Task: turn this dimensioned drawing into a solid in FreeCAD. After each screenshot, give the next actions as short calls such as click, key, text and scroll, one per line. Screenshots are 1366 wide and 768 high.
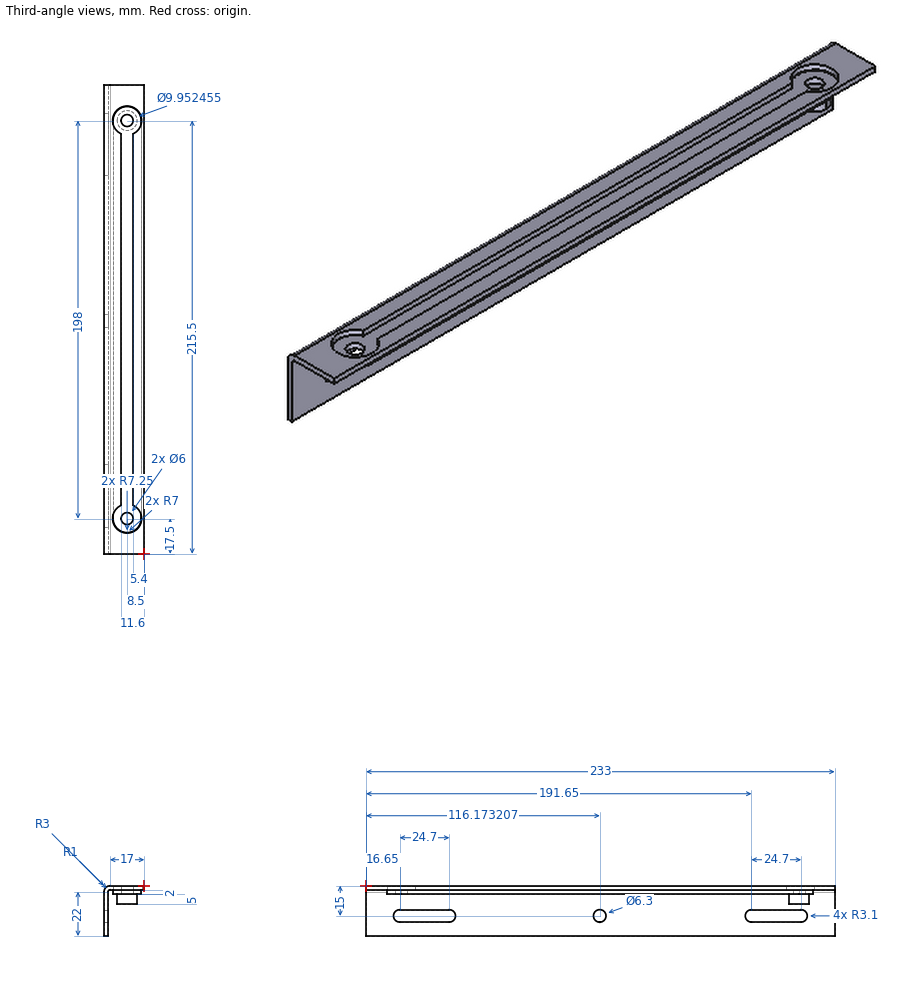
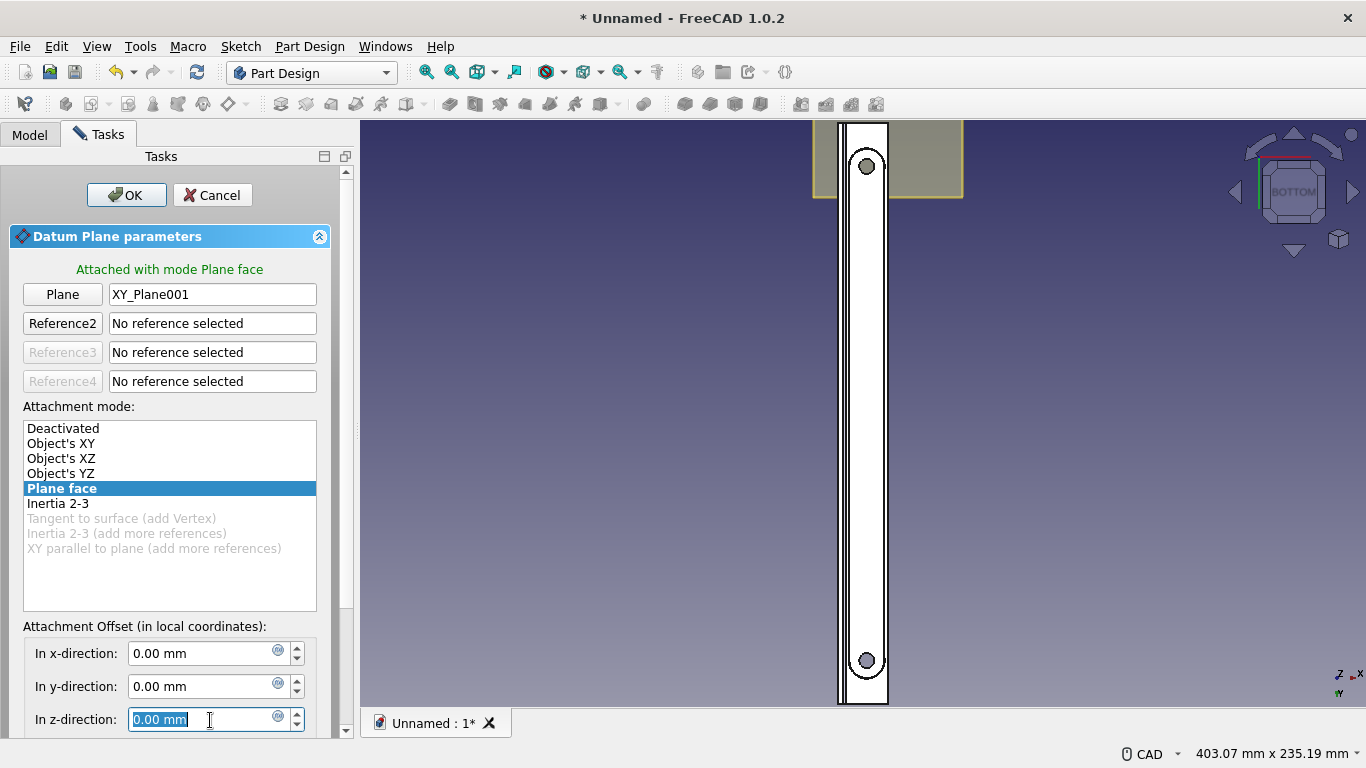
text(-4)
key(Tab)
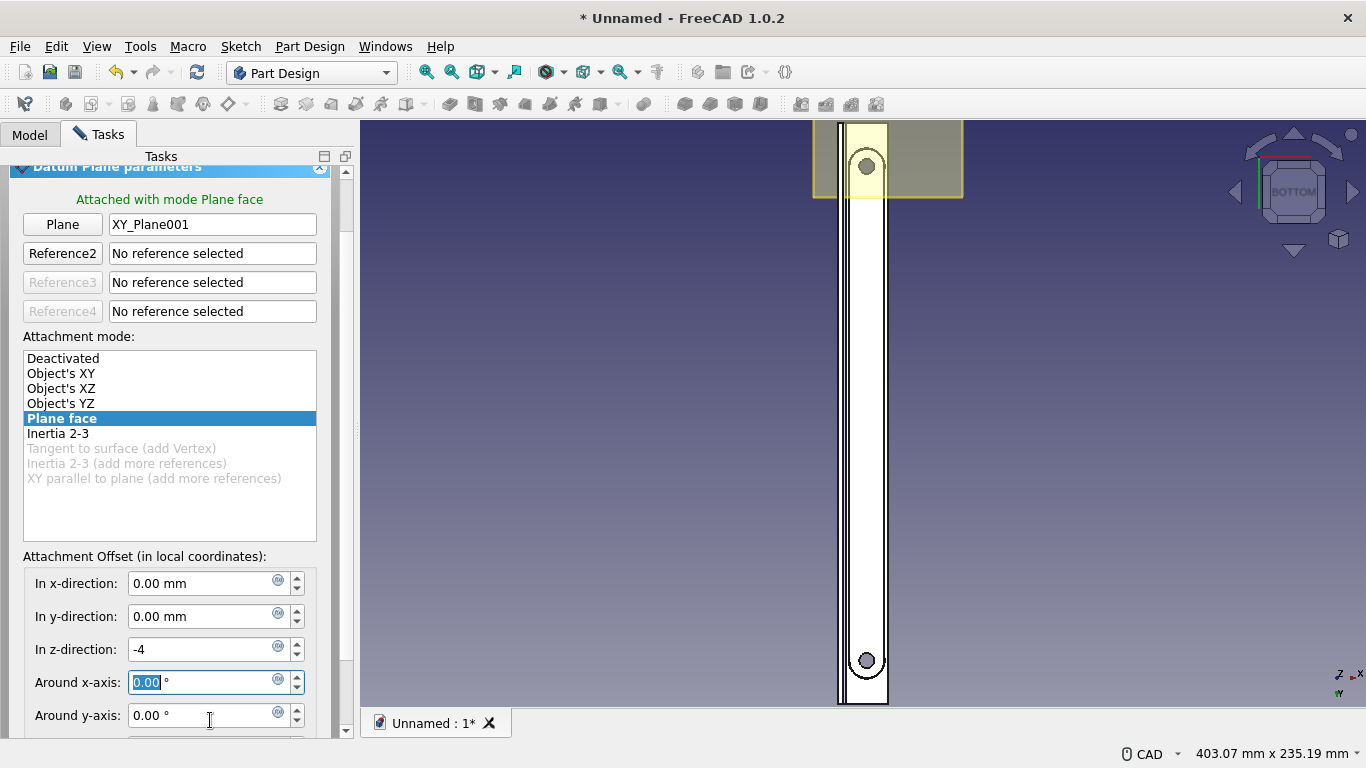
scroll(346, 452, up, 2)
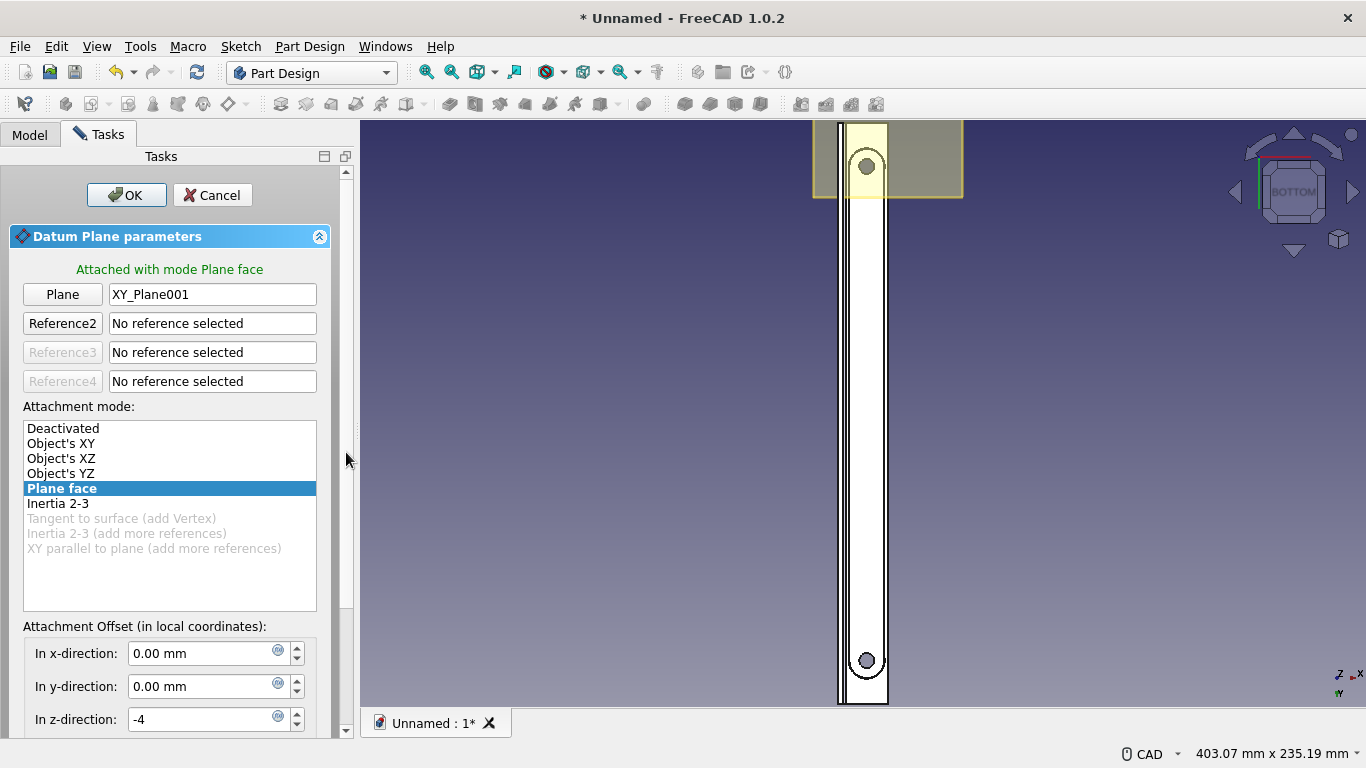
click(127, 195)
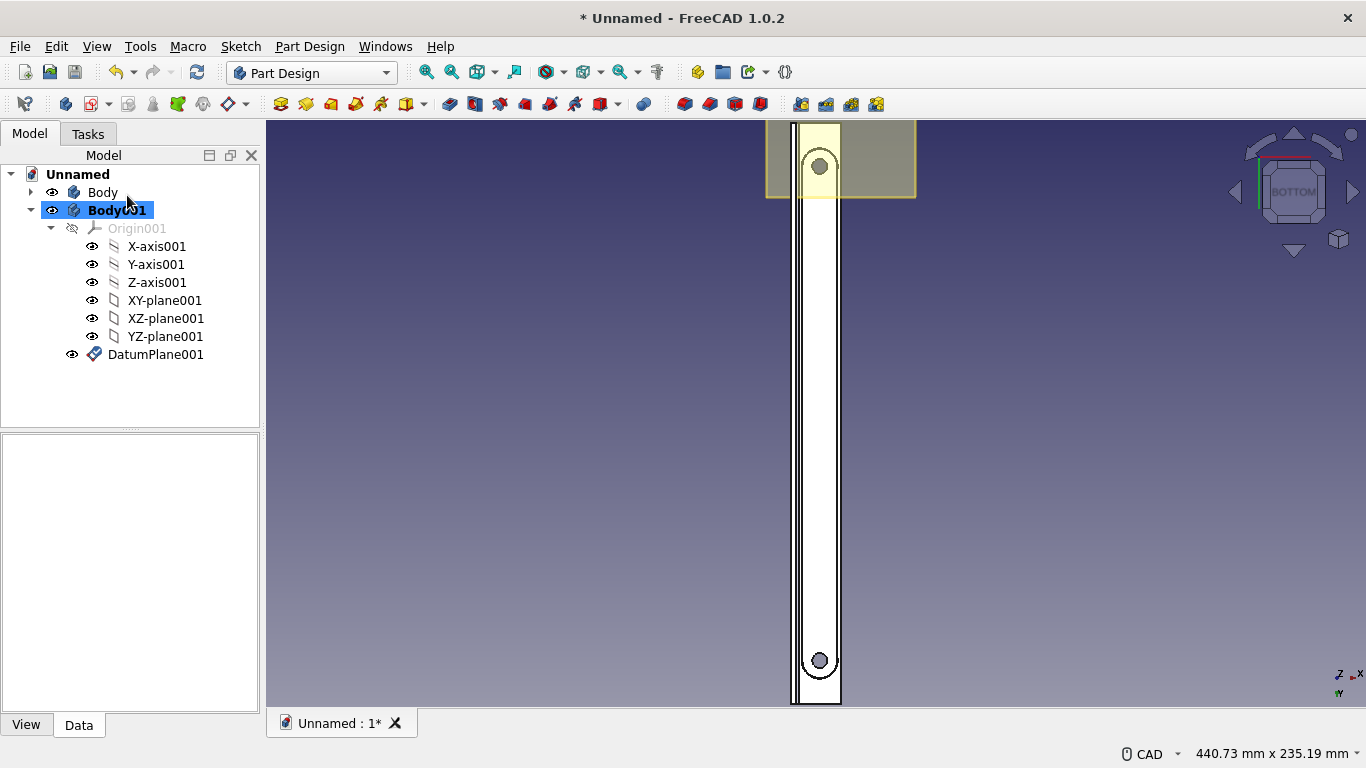
click(117, 354)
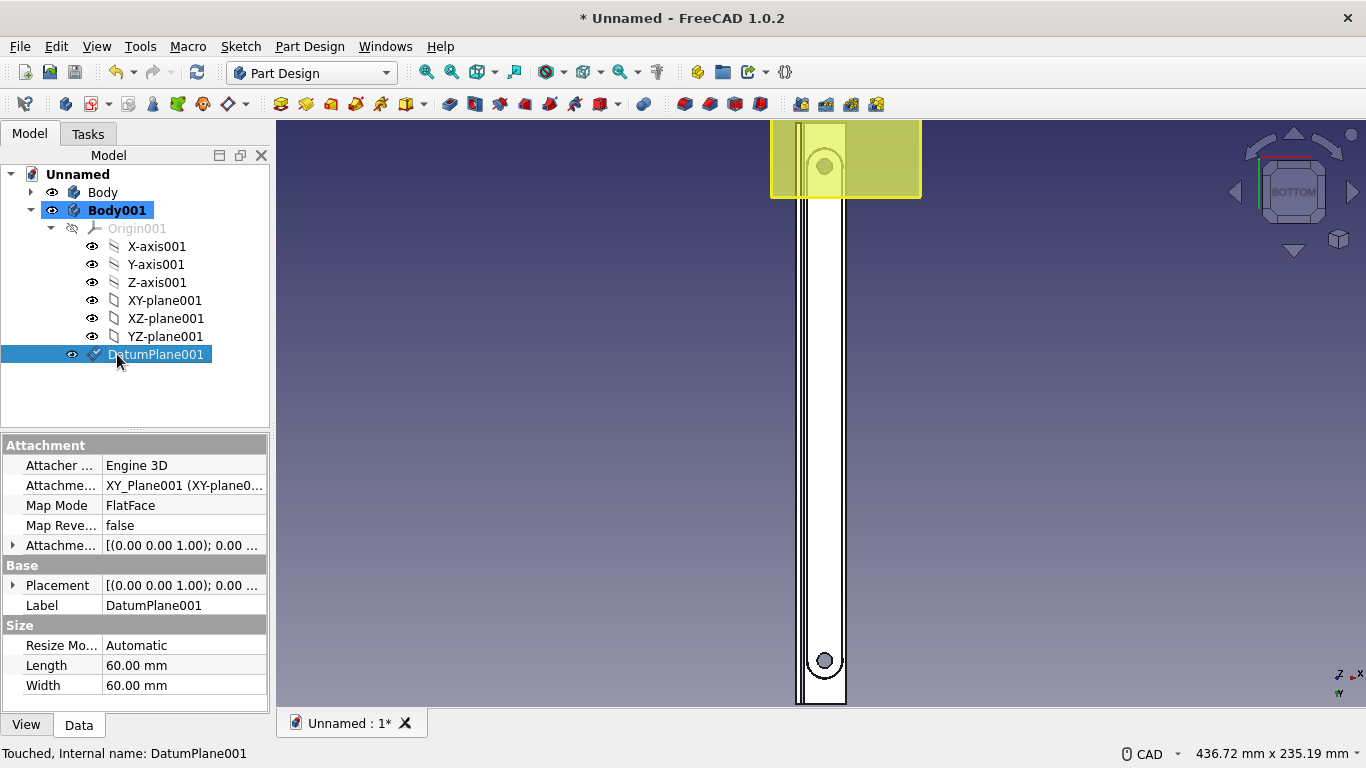
click(90, 104)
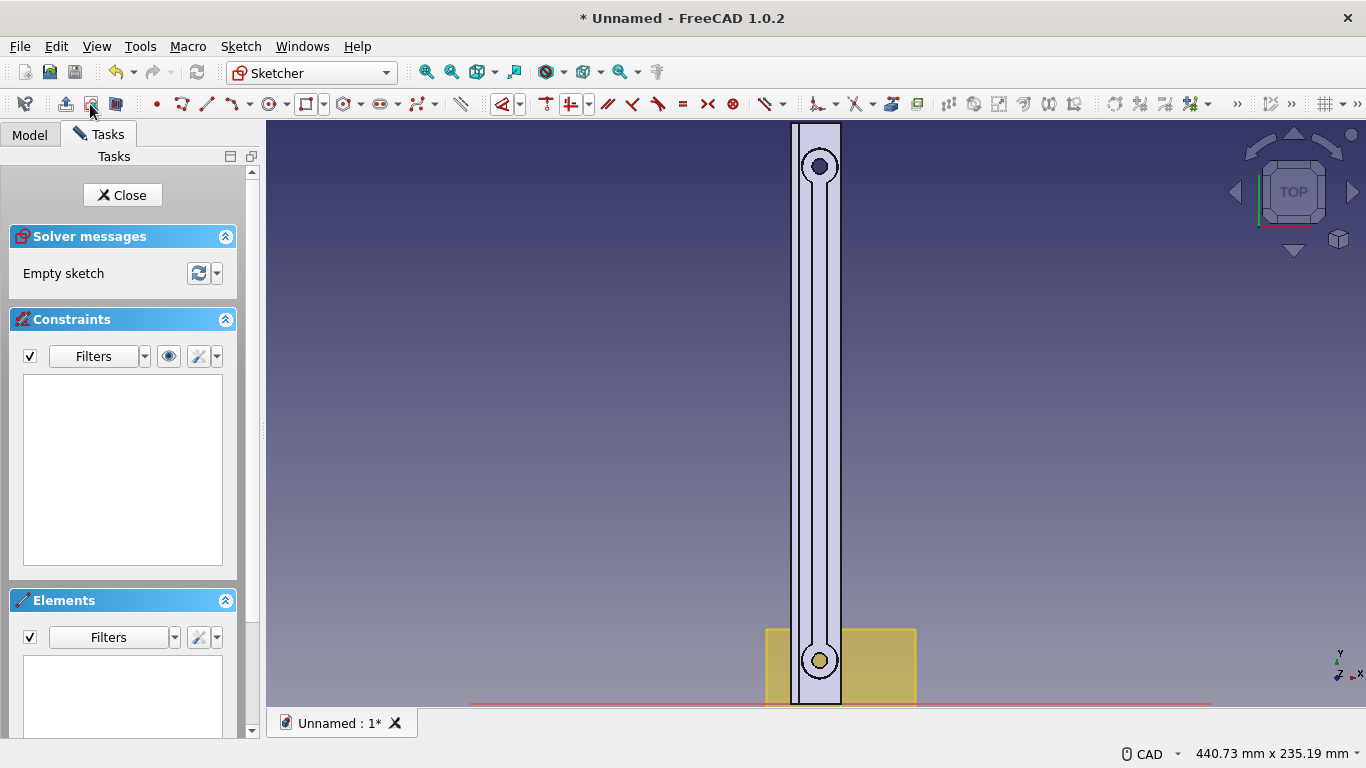
scroll(824, 150, up, 14)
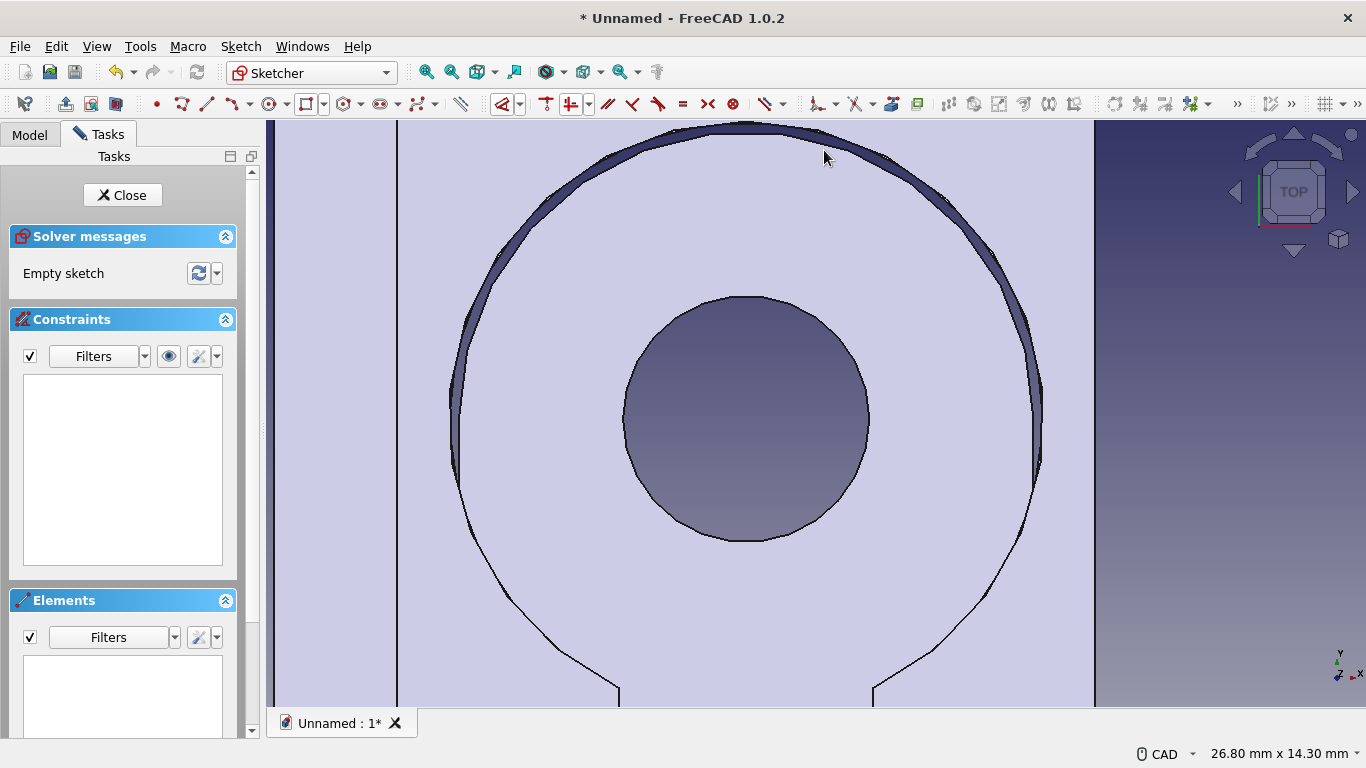
click(268, 104)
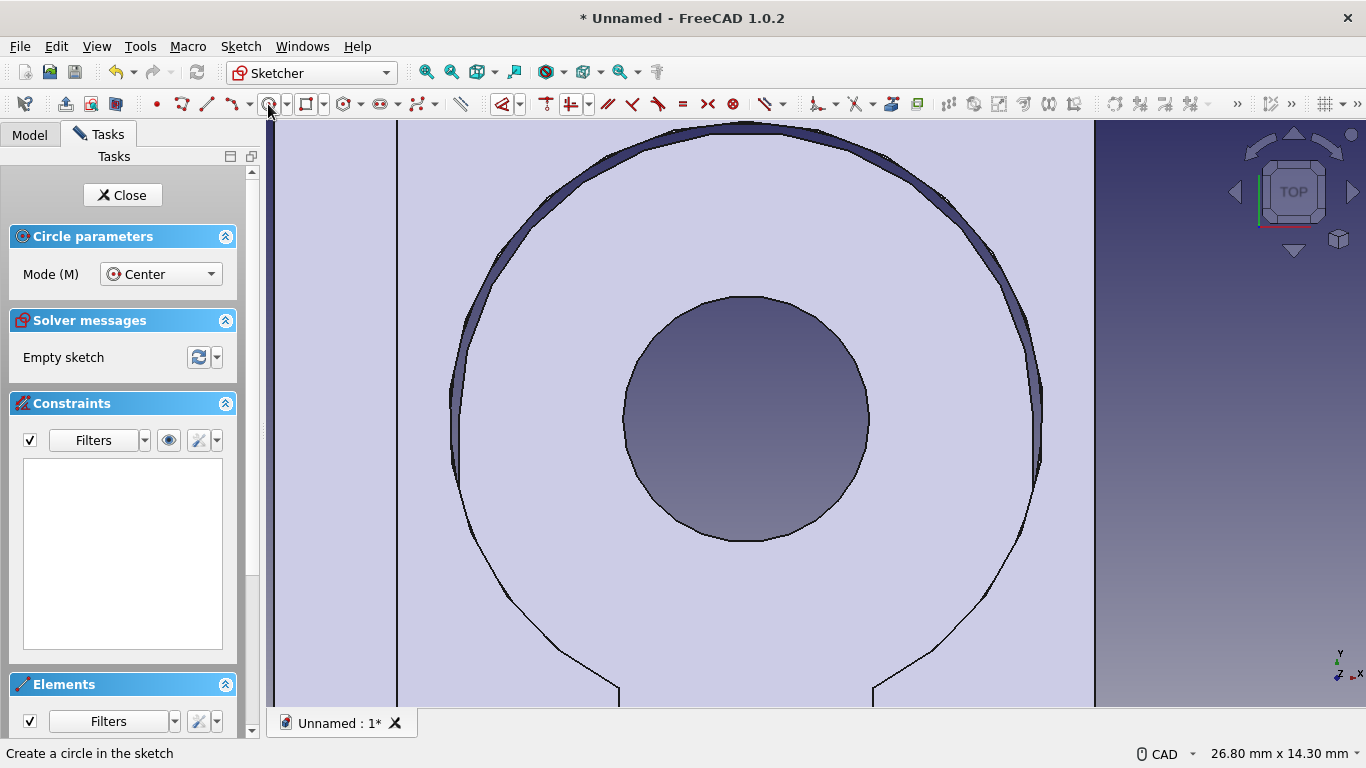
click(746, 419)
click(891, 275)
key(Escape)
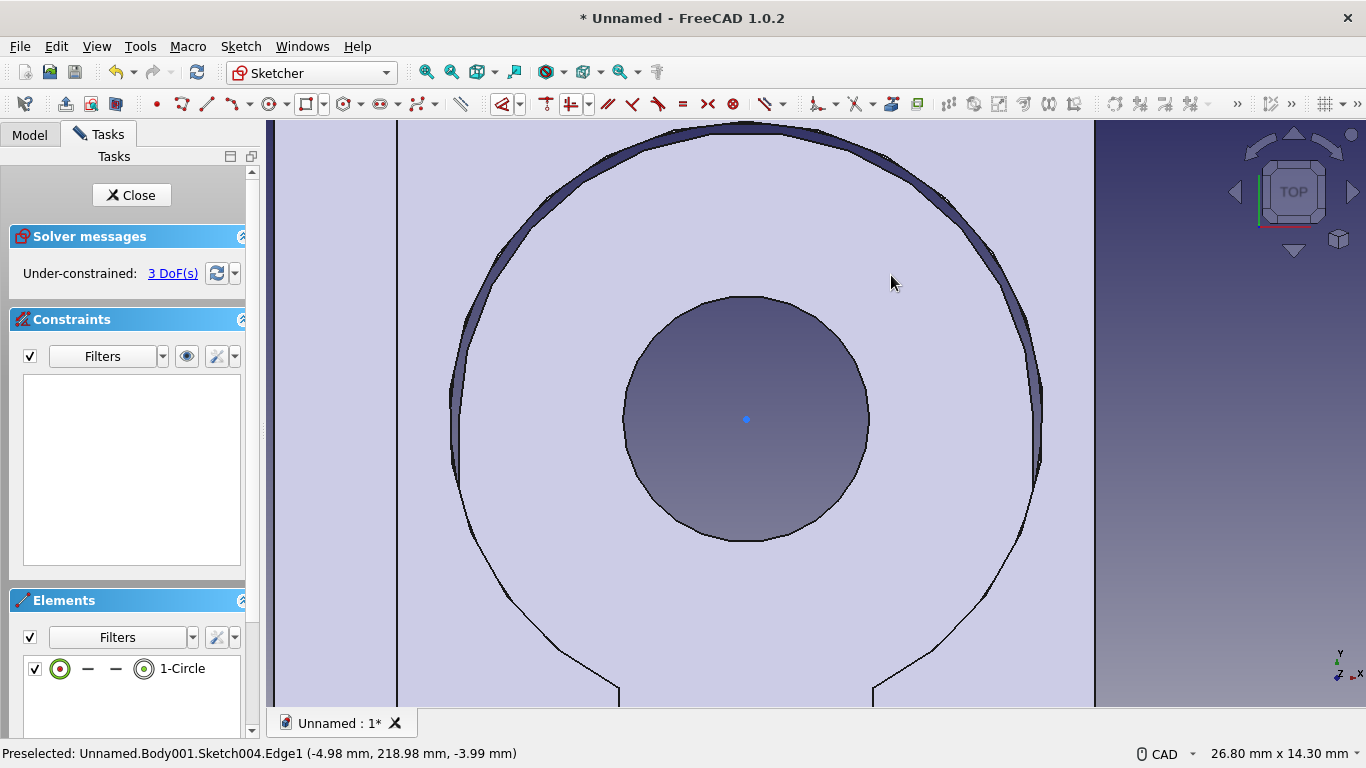
click(890, 275)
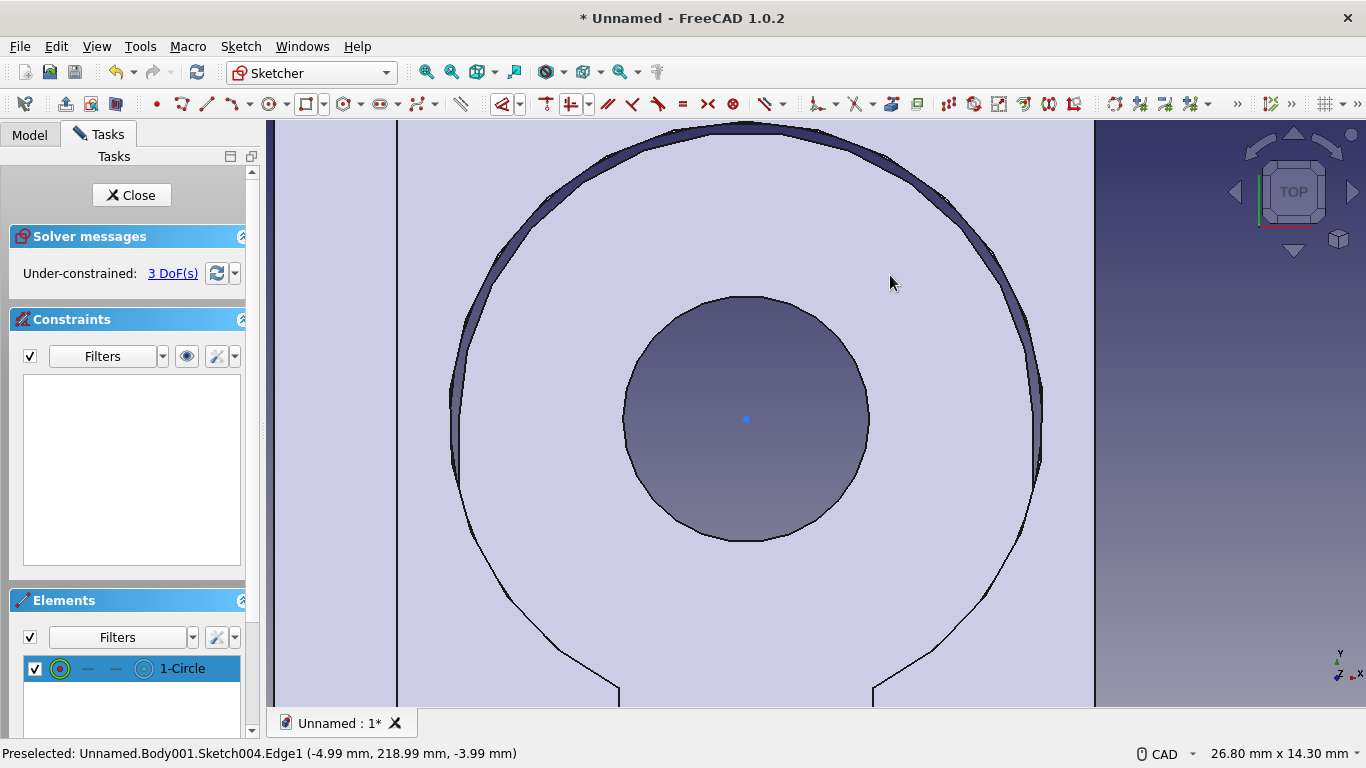
key(k)
key(o)